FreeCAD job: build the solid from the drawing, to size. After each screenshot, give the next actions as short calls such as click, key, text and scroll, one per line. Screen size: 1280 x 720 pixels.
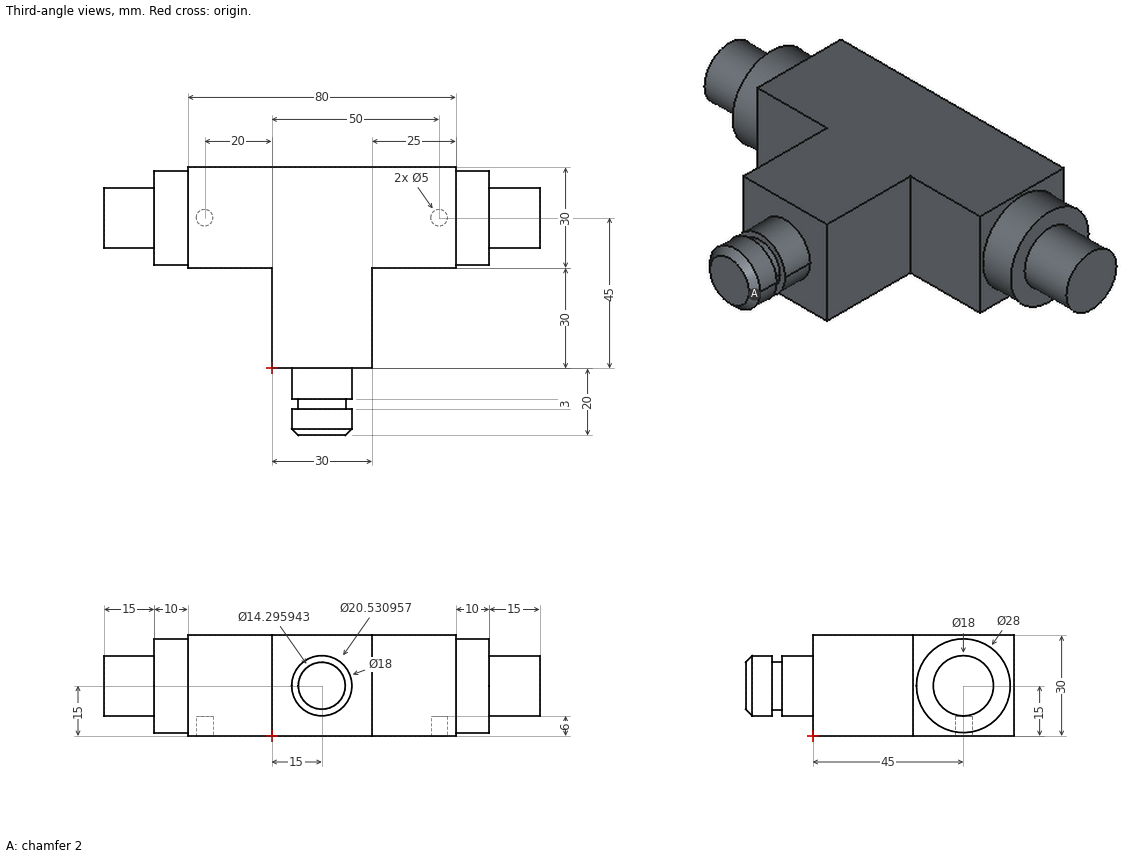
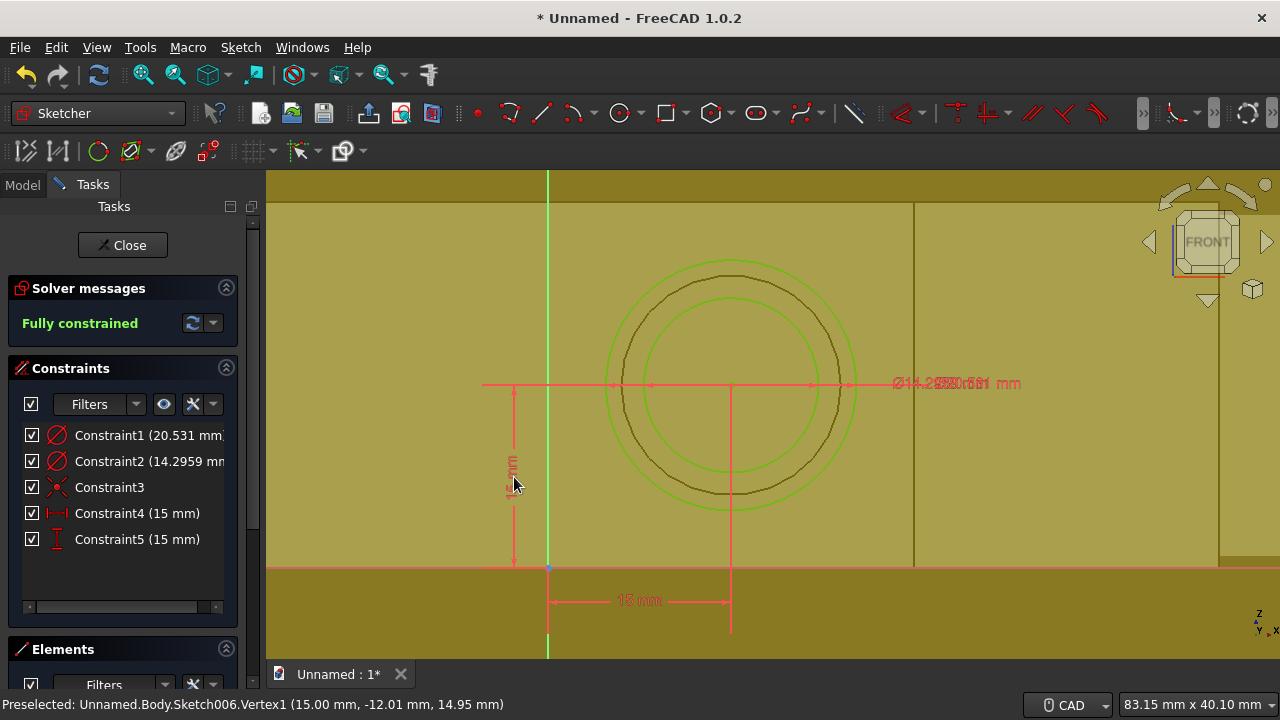
click(123, 245)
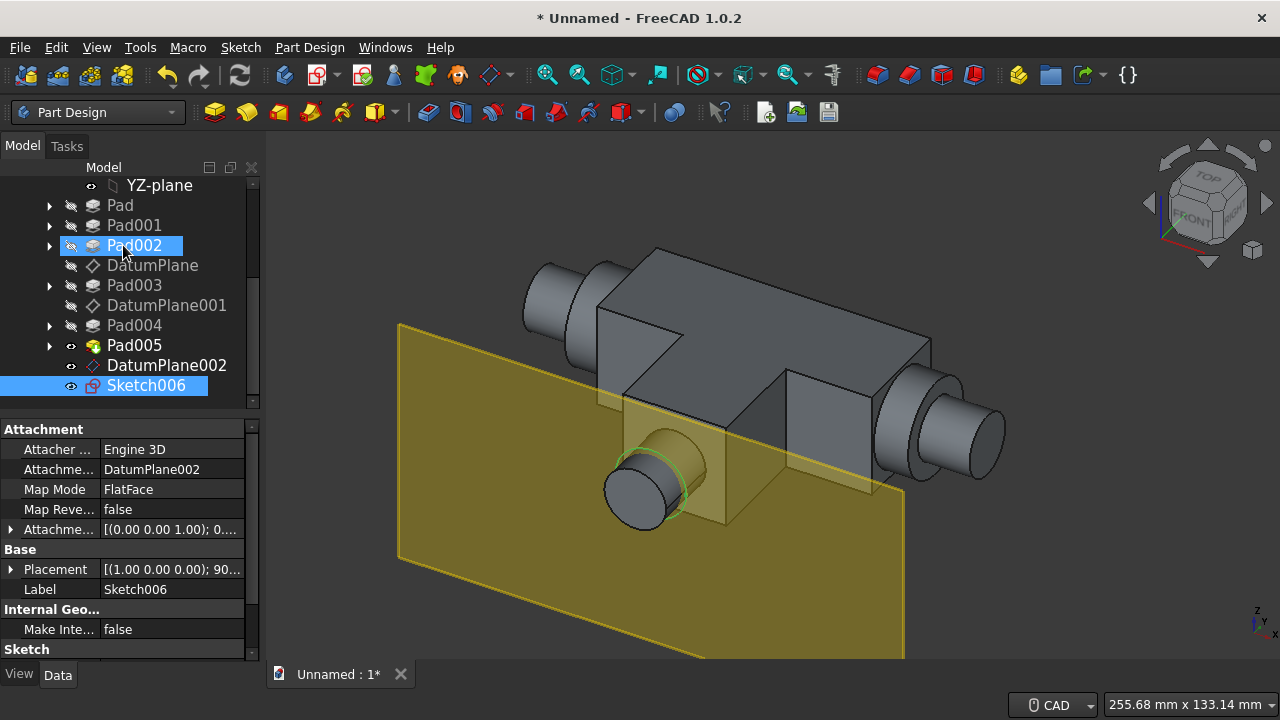
click(430, 112)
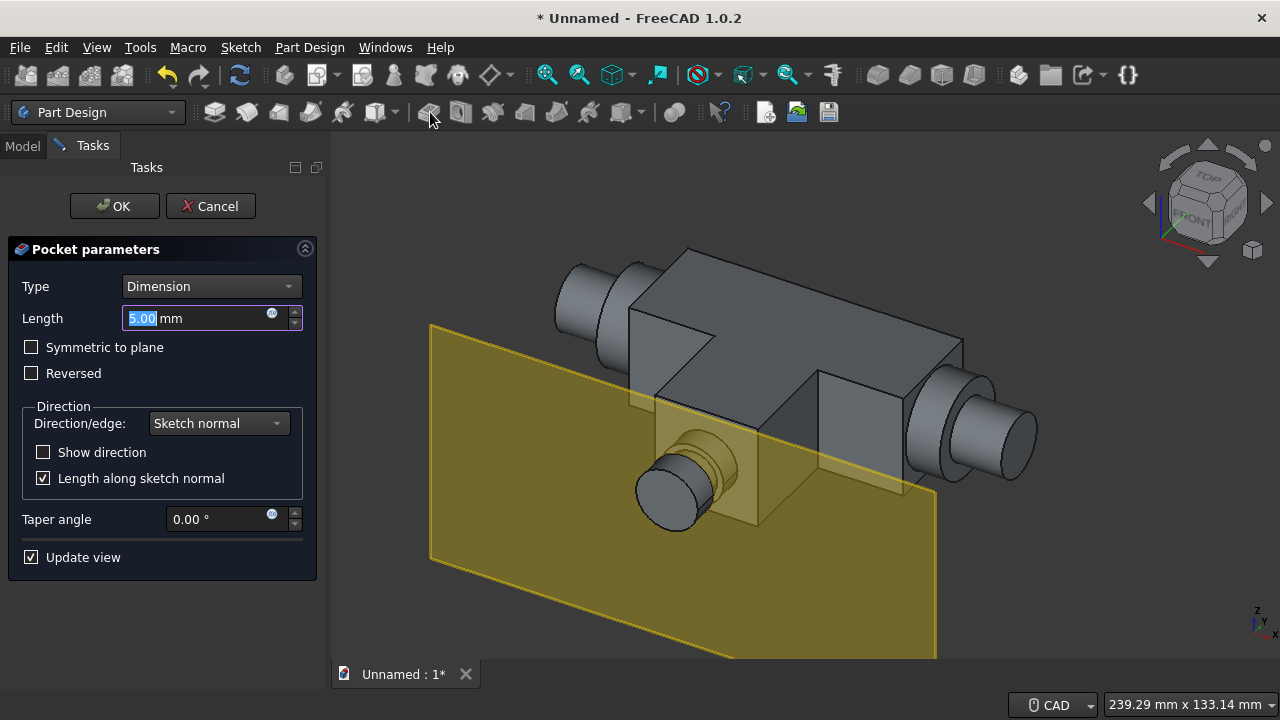
text(3)
key(Tab)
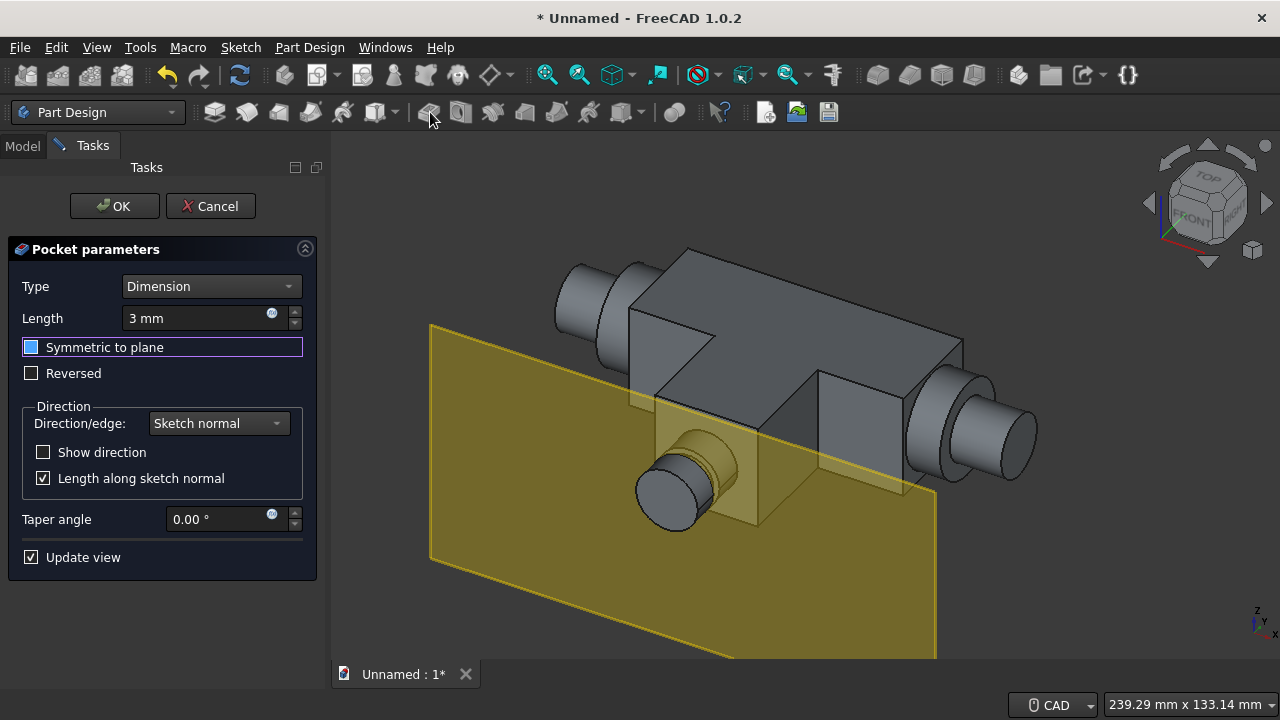
click(115, 206)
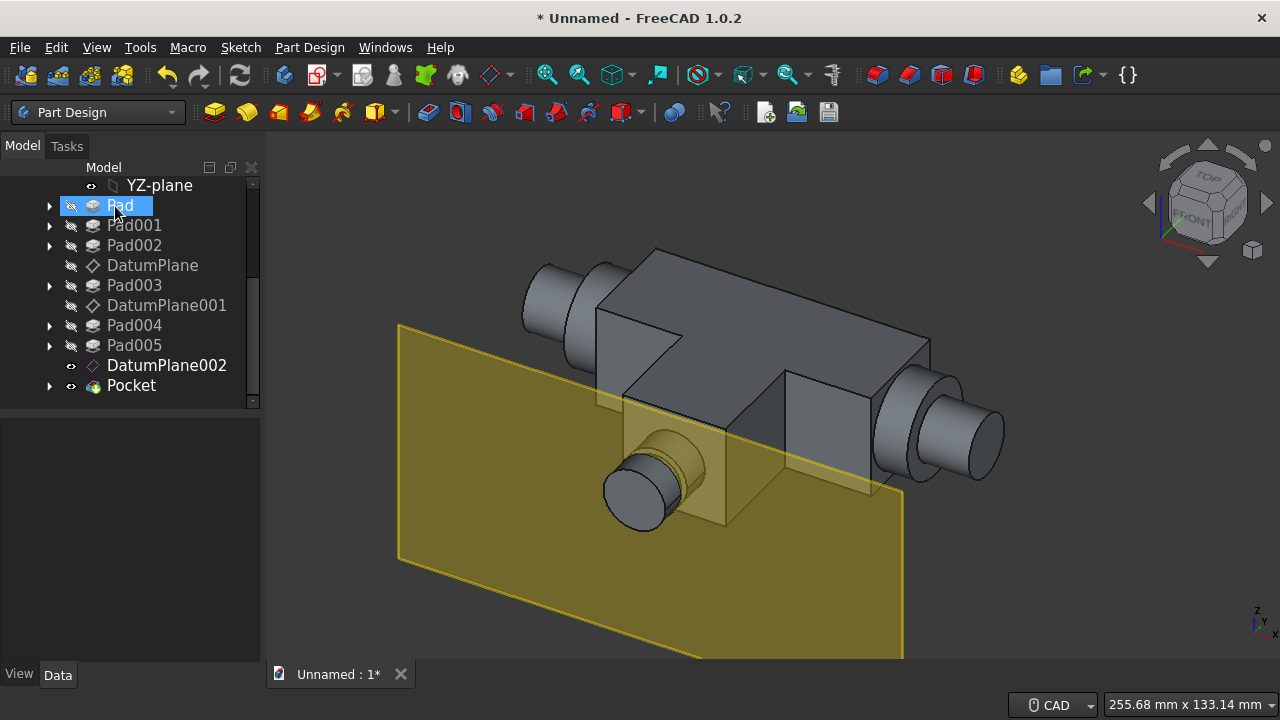
click(116, 366)
key(space)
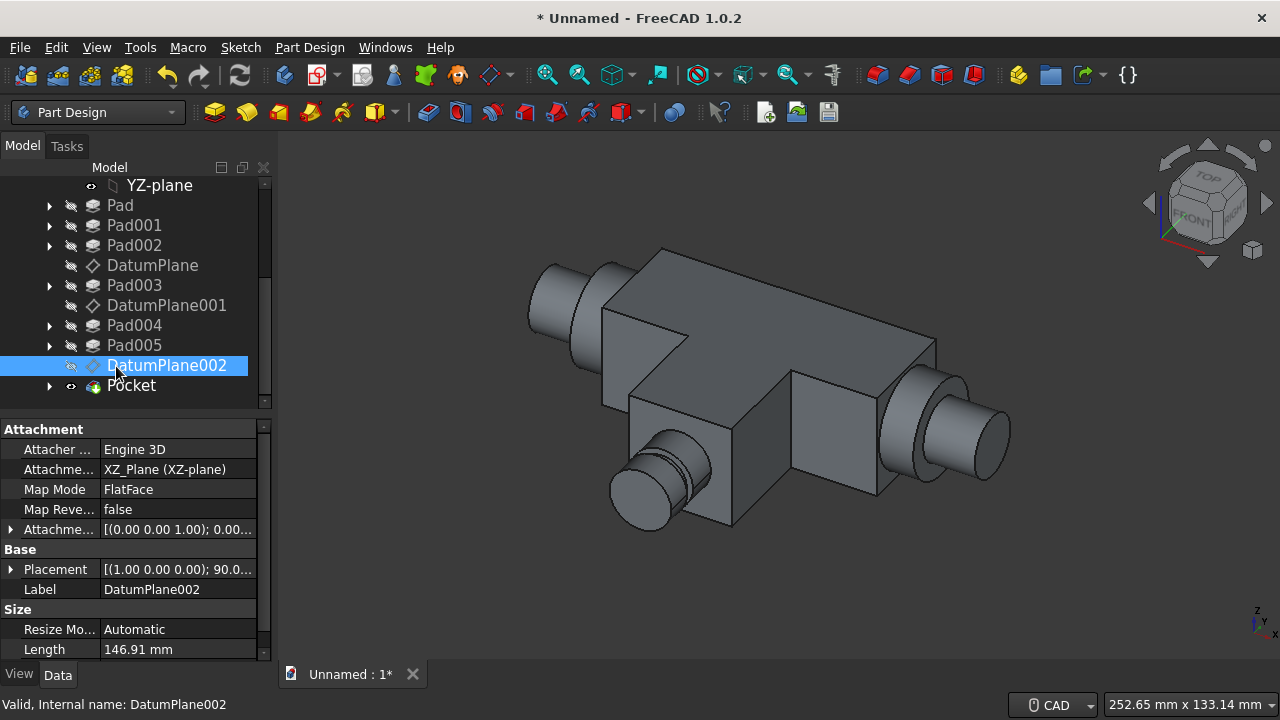
click(615, 474)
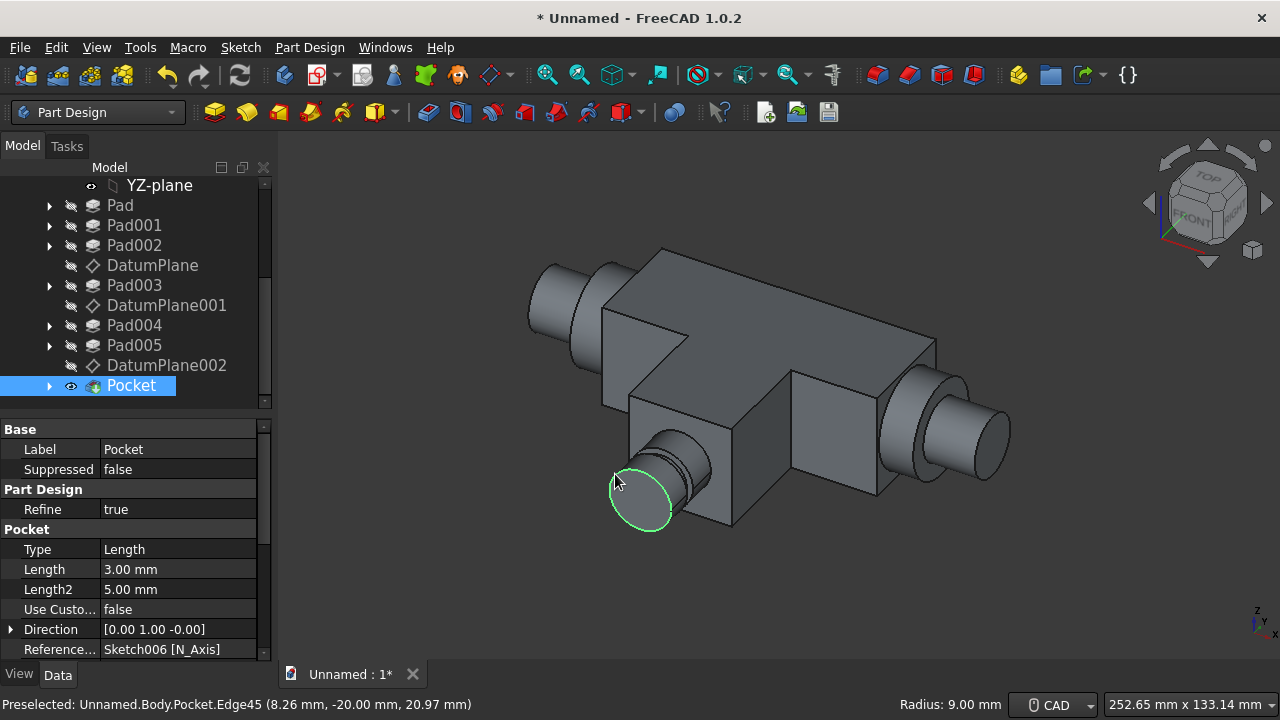
click(910, 76)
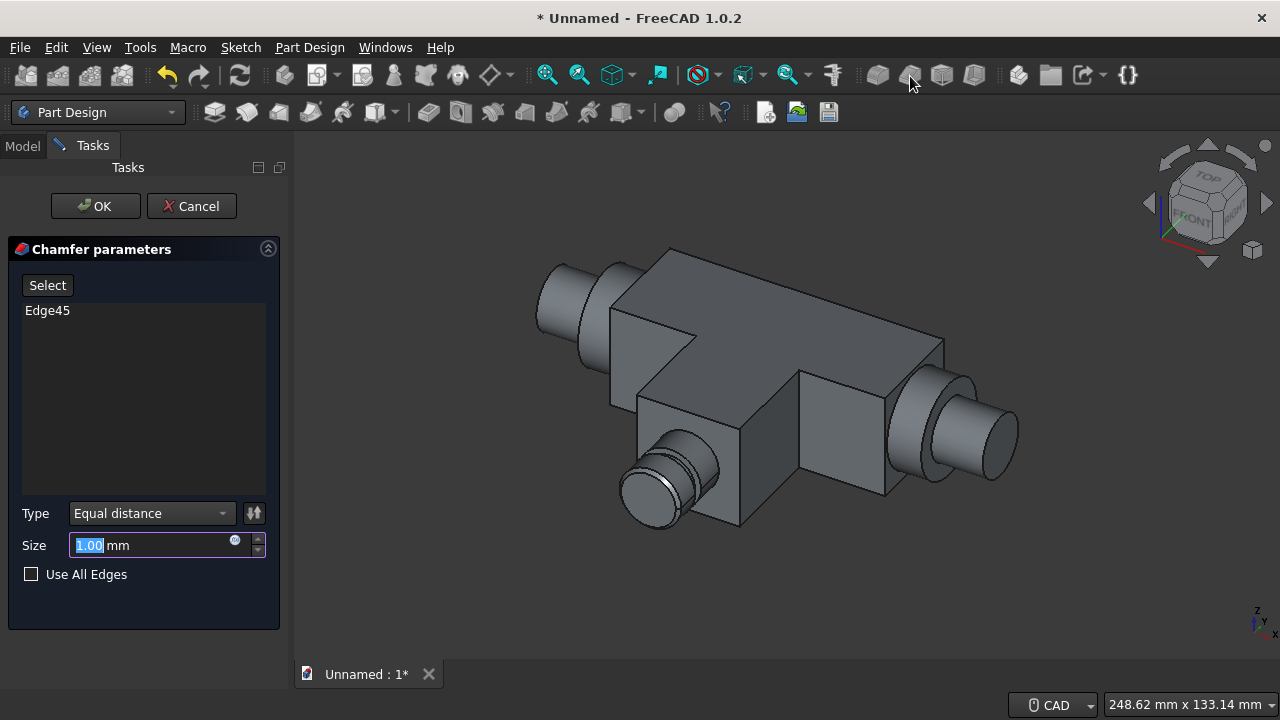
text(2)
key(Tab)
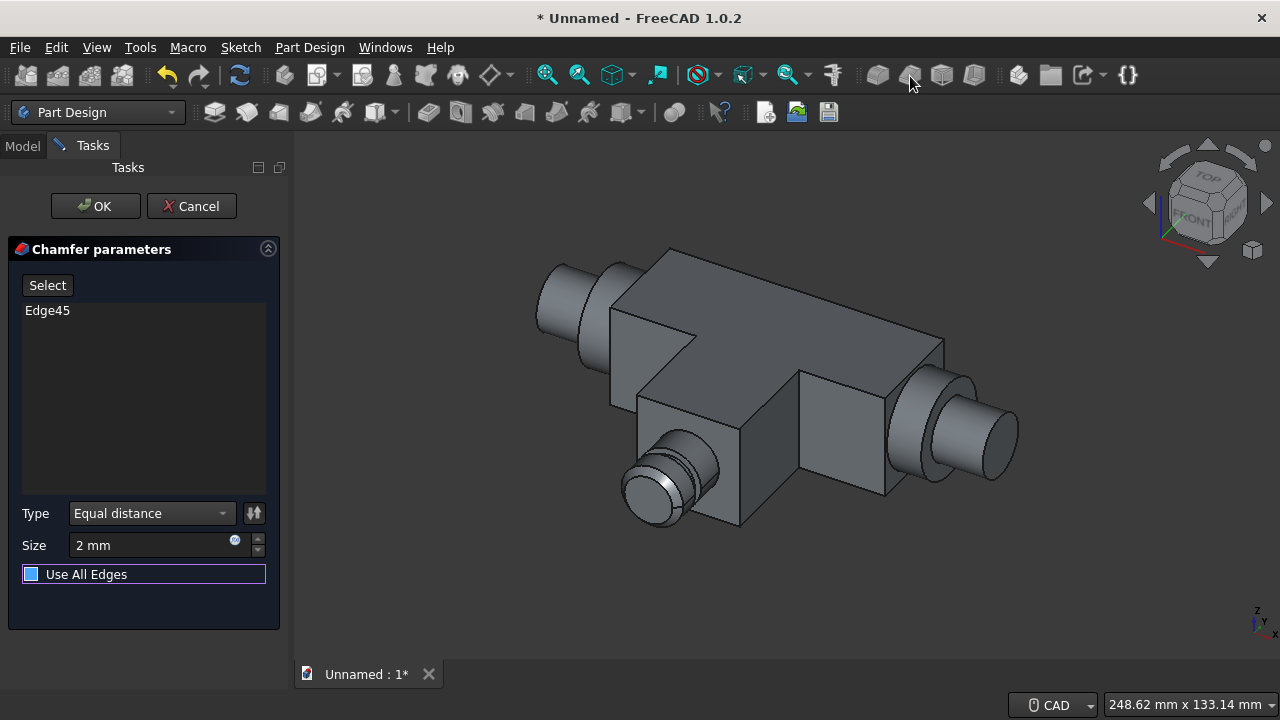
click(96, 206)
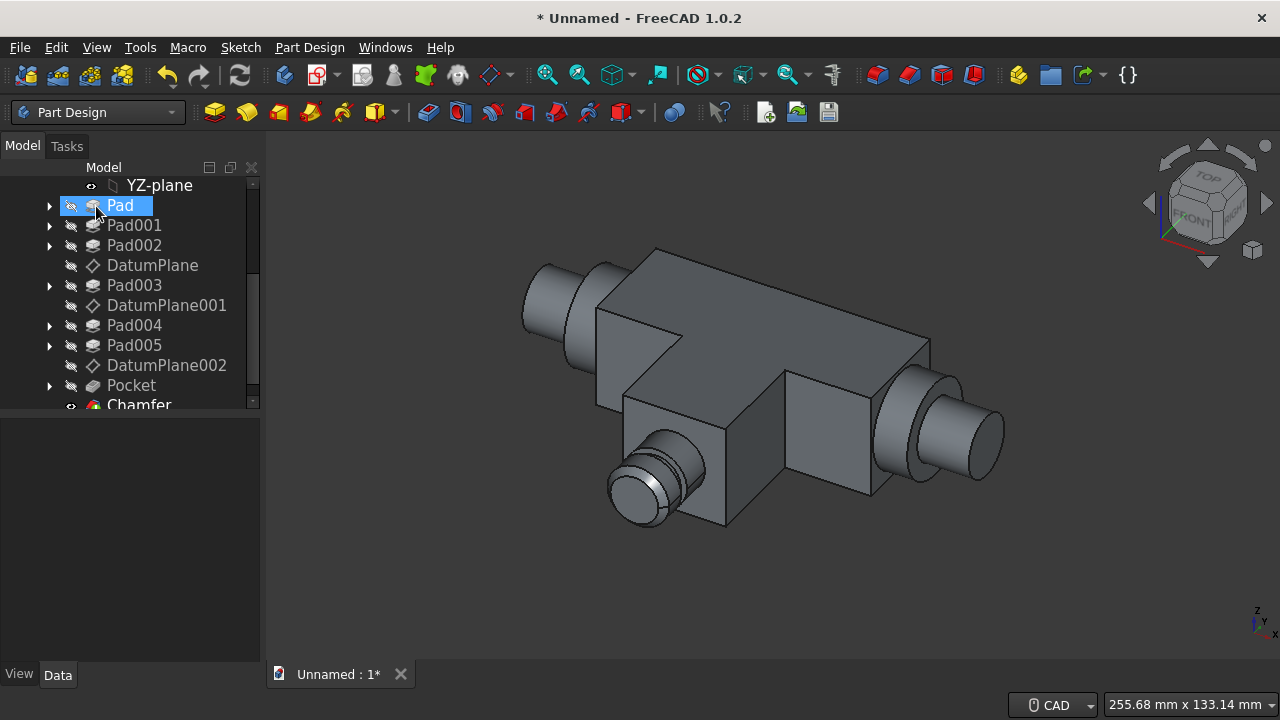
click(318, 76)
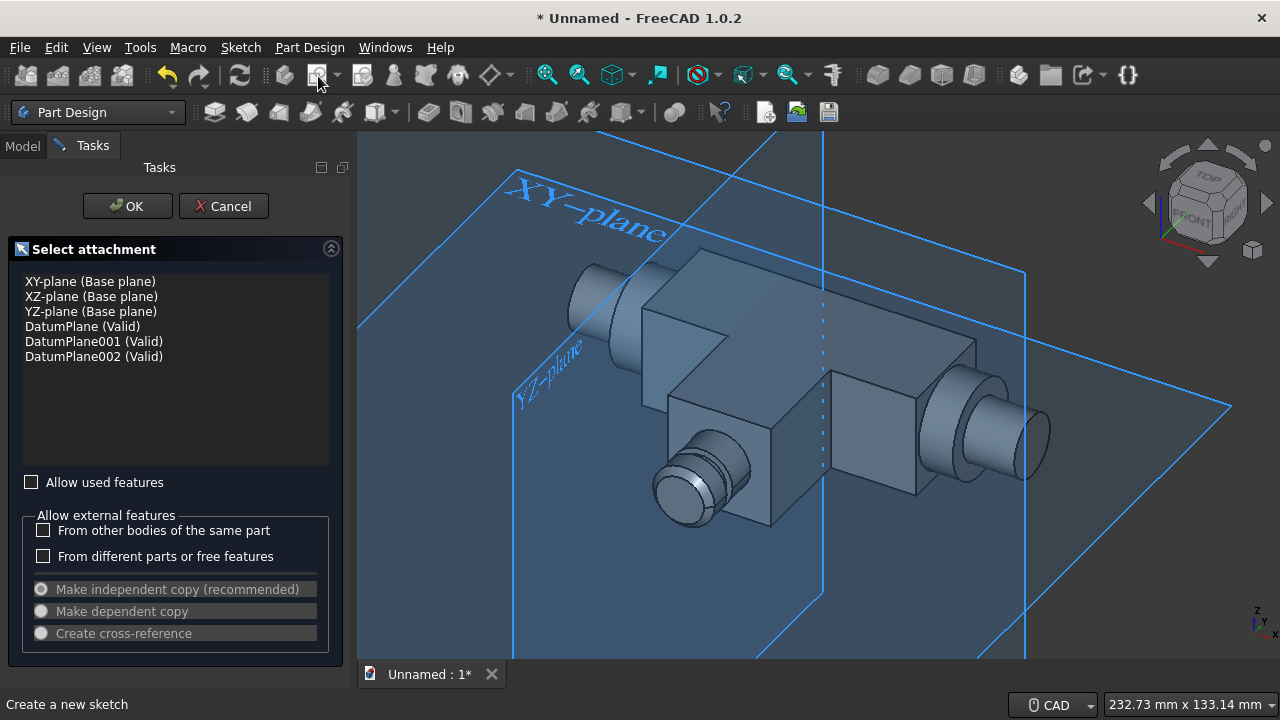
click(82, 282)